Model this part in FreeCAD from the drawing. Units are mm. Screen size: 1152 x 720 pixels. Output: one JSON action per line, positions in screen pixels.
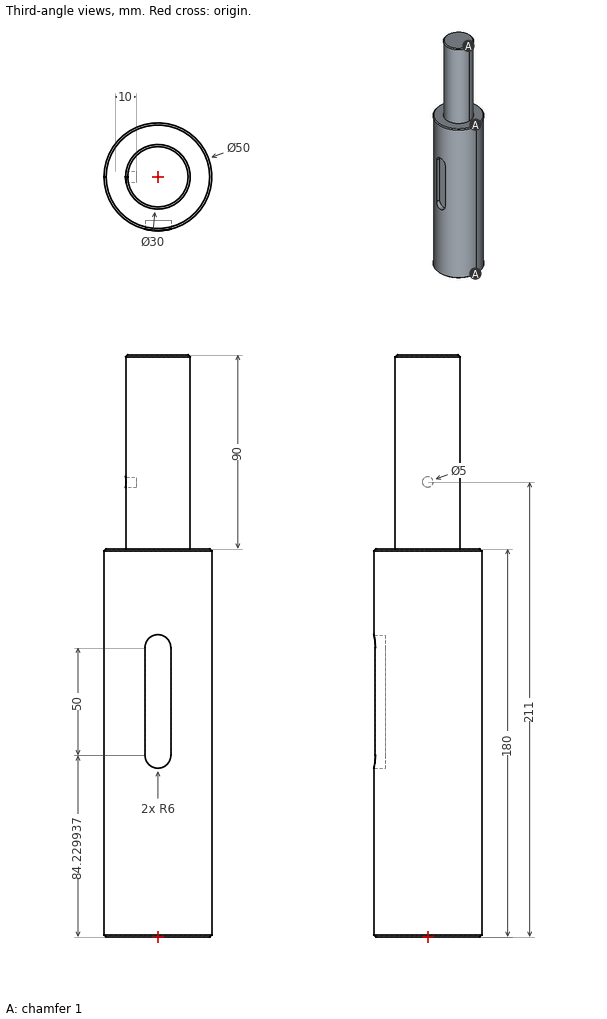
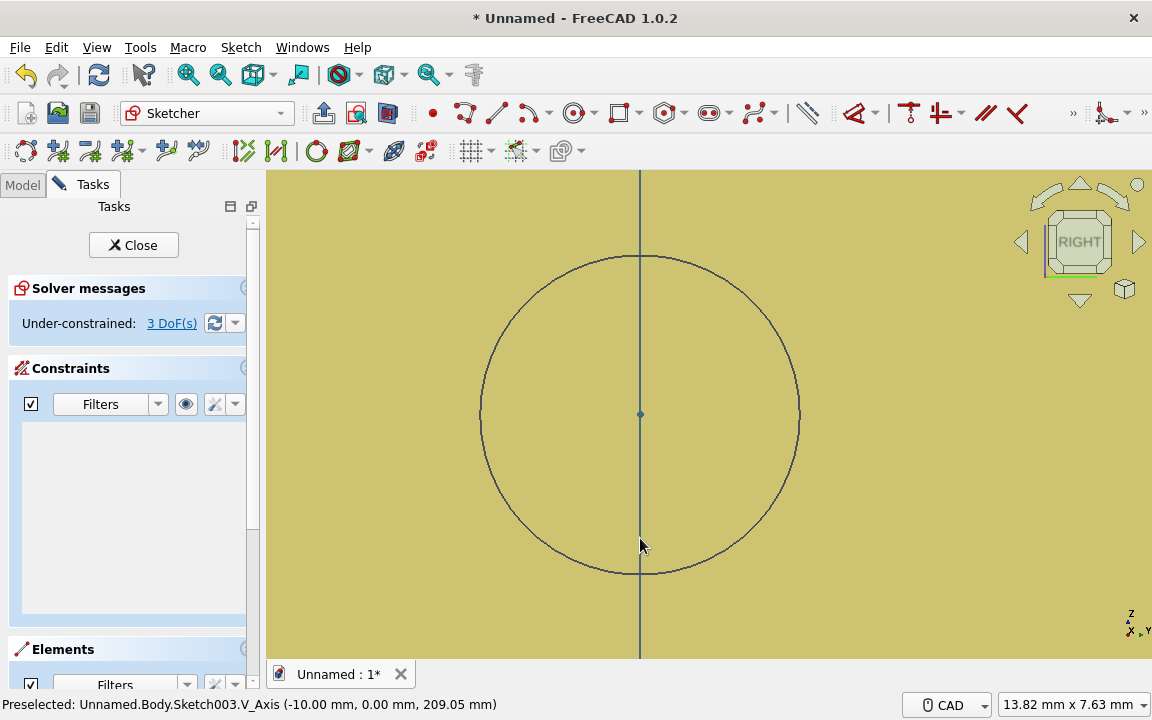
{"action": "left_click", "coordinate": [910, 114]}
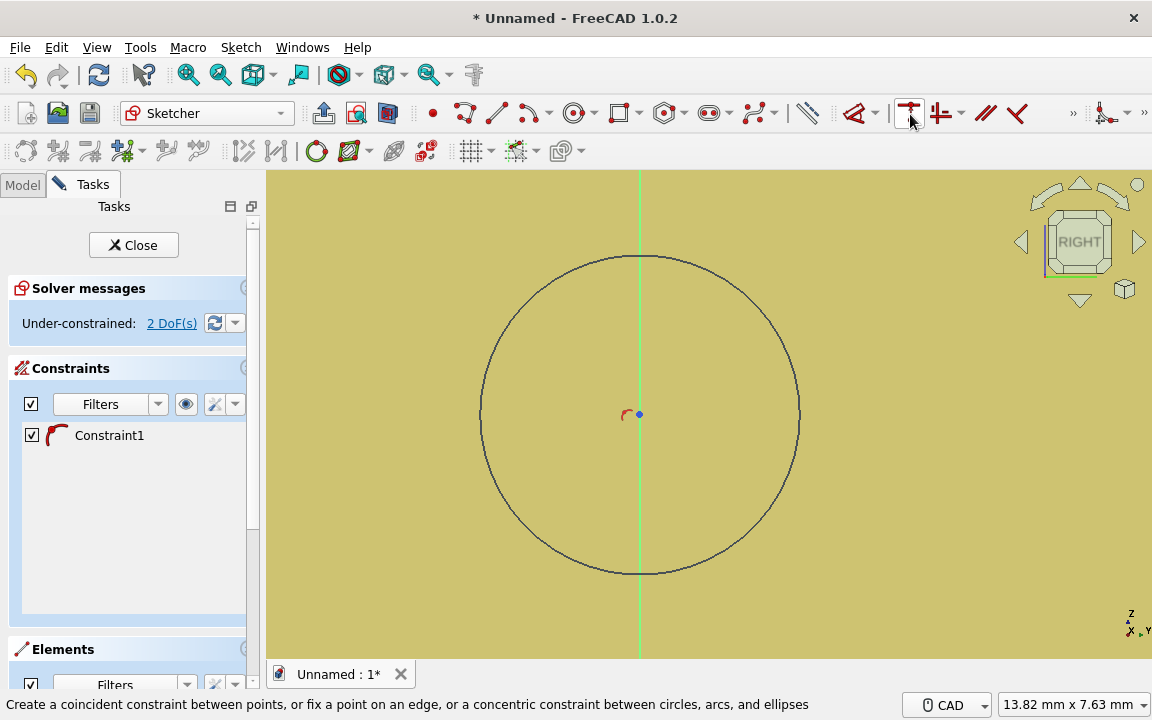
{"action": "key", "text": "d"}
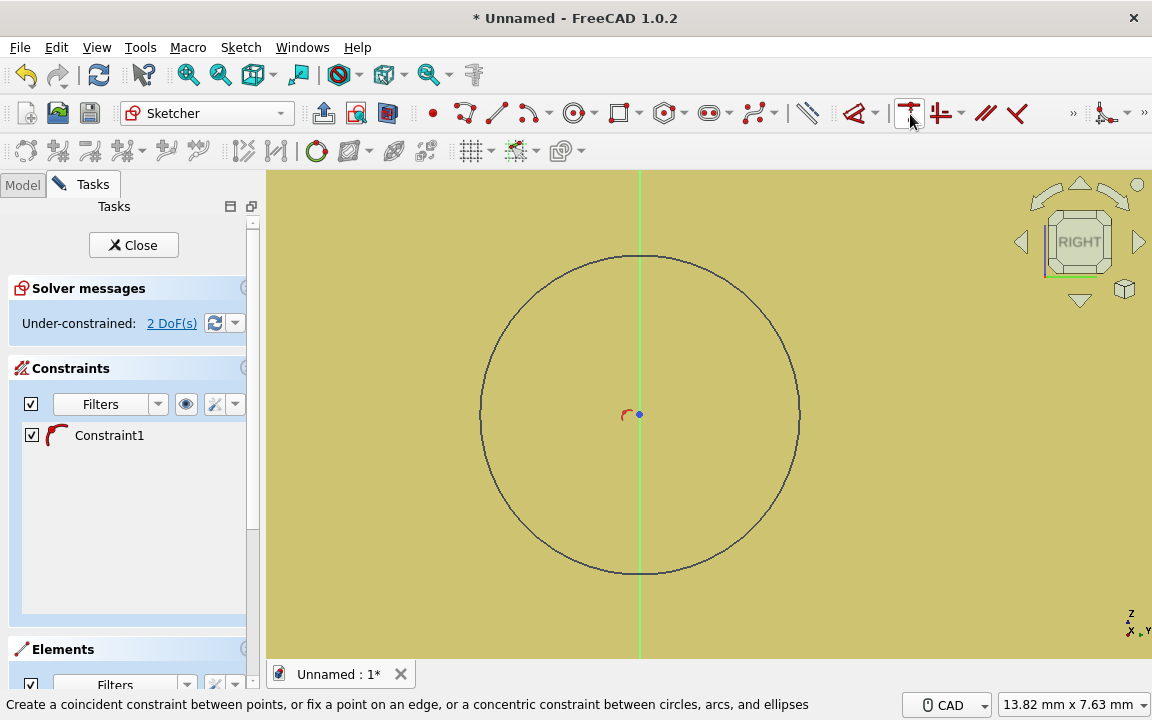
{"action": "left_click", "coordinate": [753, 302]}
{"action": "left_click", "coordinate": [776, 279]}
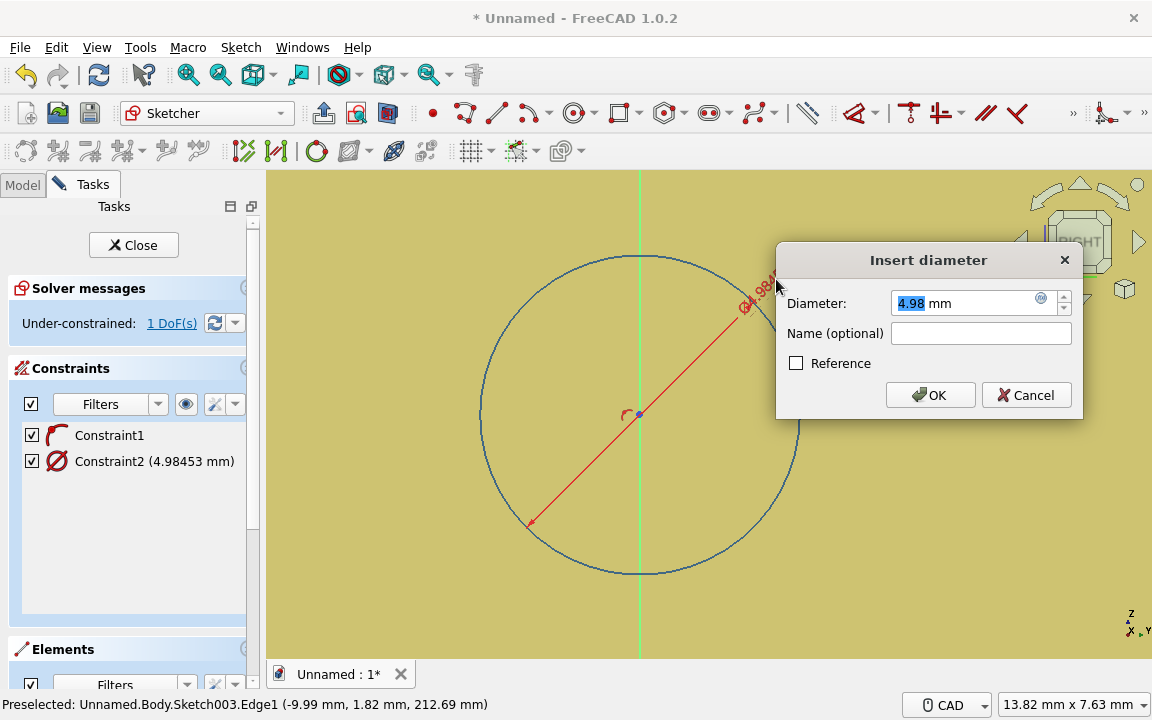
{"action": "type", "text": "5"}
{"action": "key", "text": "Return"}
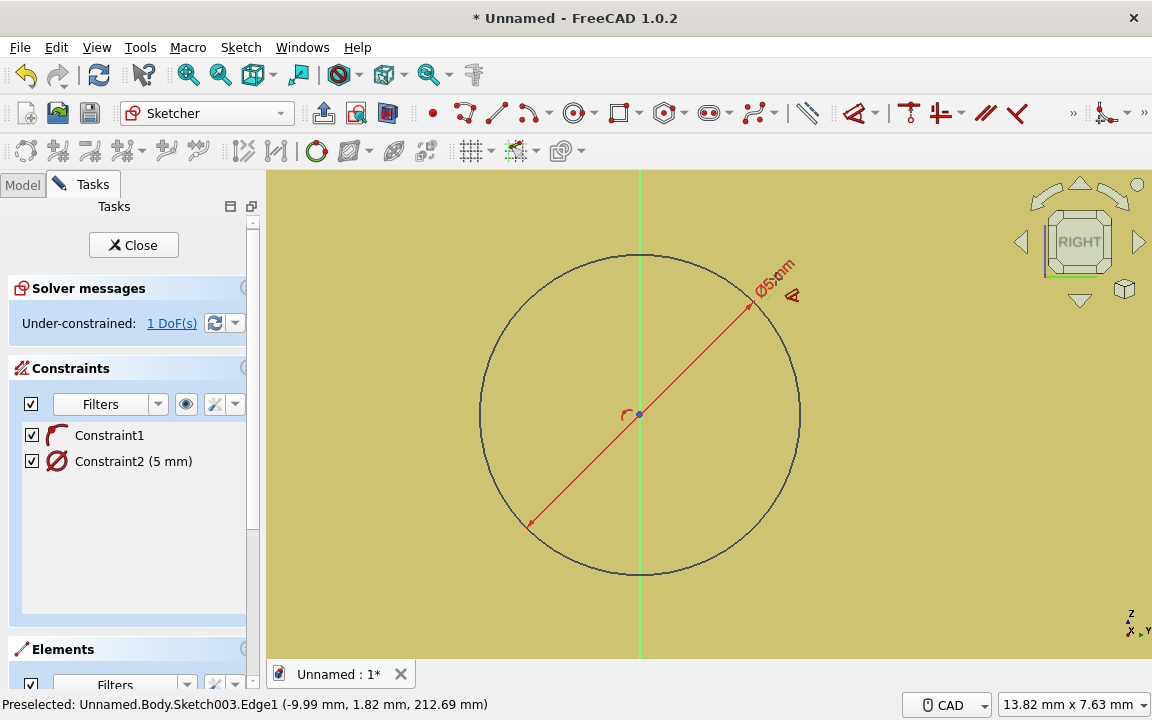
{"action": "left_click", "coordinate": [640, 415]}
{"action": "left_click", "coordinate": [674, 523]}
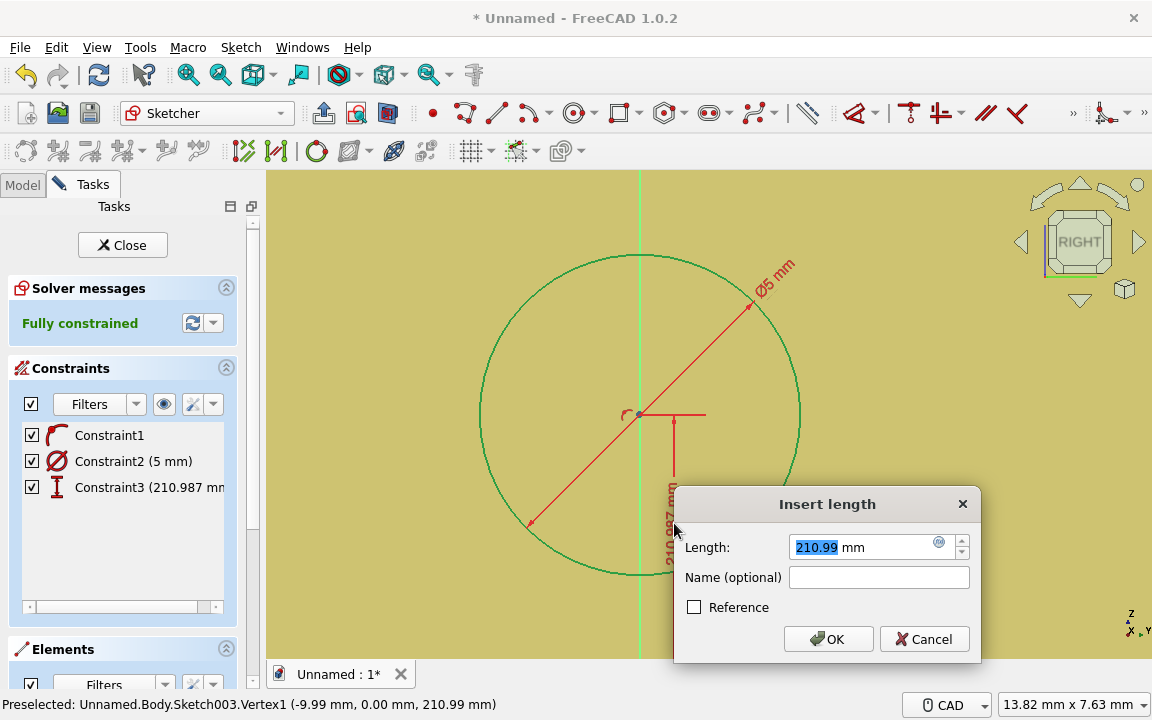
{"action": "type", "text": "211"}
{"action": "key", "text": "Return"}
{"action": "key", "text": "Escape"}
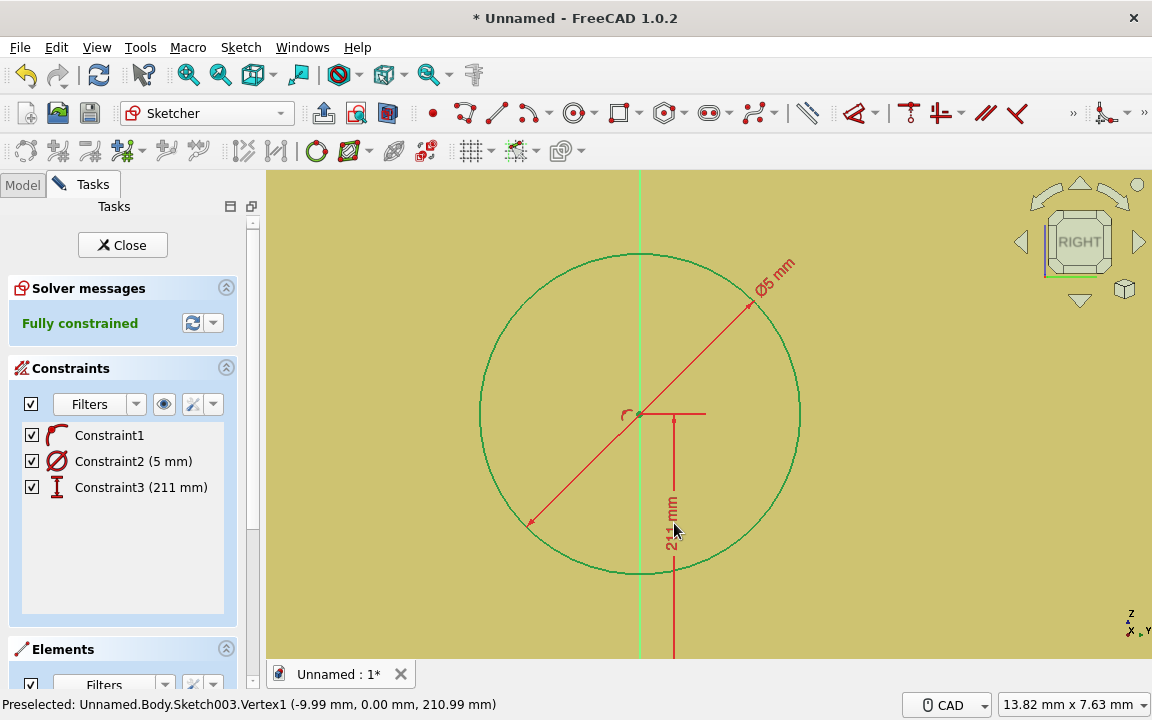
{"action": "left_click", "coordinate": [123, 245]}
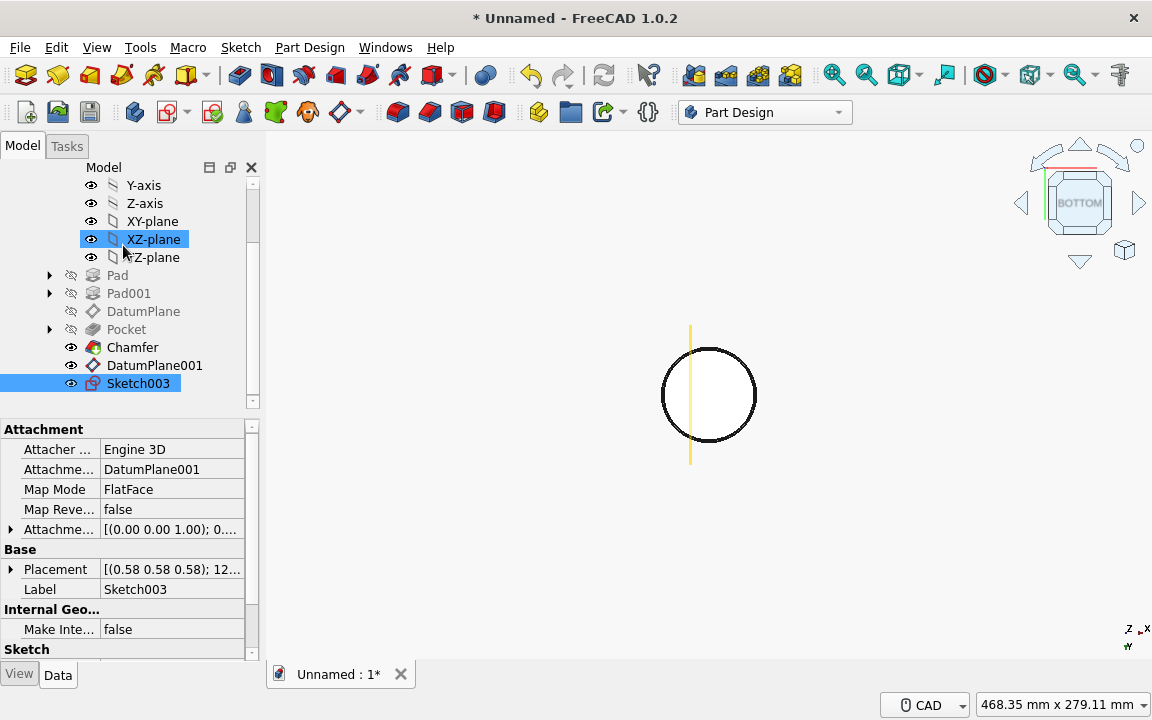
{"action": "left_click", "coordinate": [240, 76]}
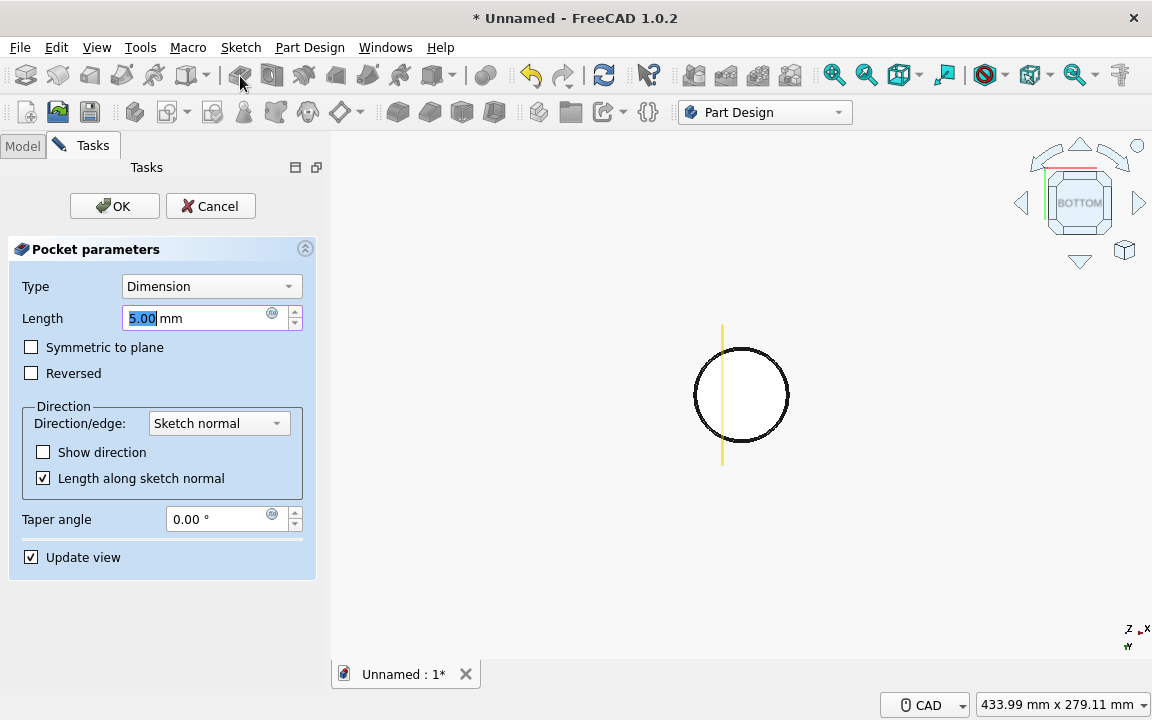
{"action": "type", "text": "10"}
{"action": "key", "text": "Tab"}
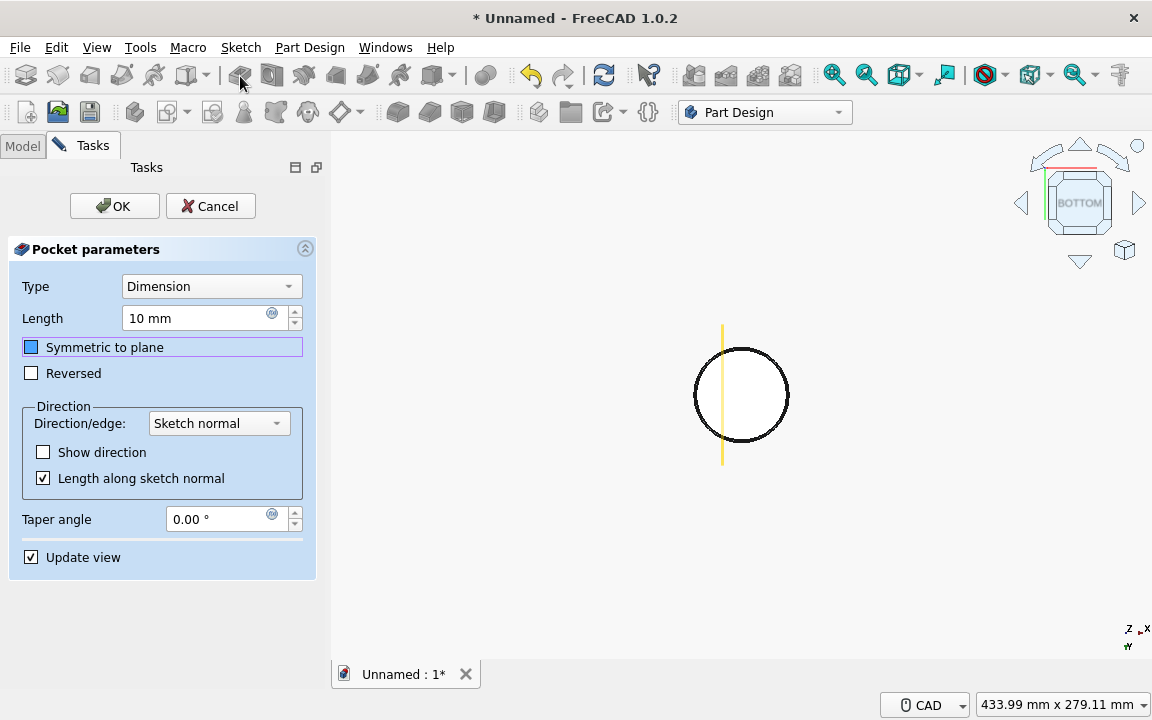
{"action": "left_click", "coordinate": [115, 206]}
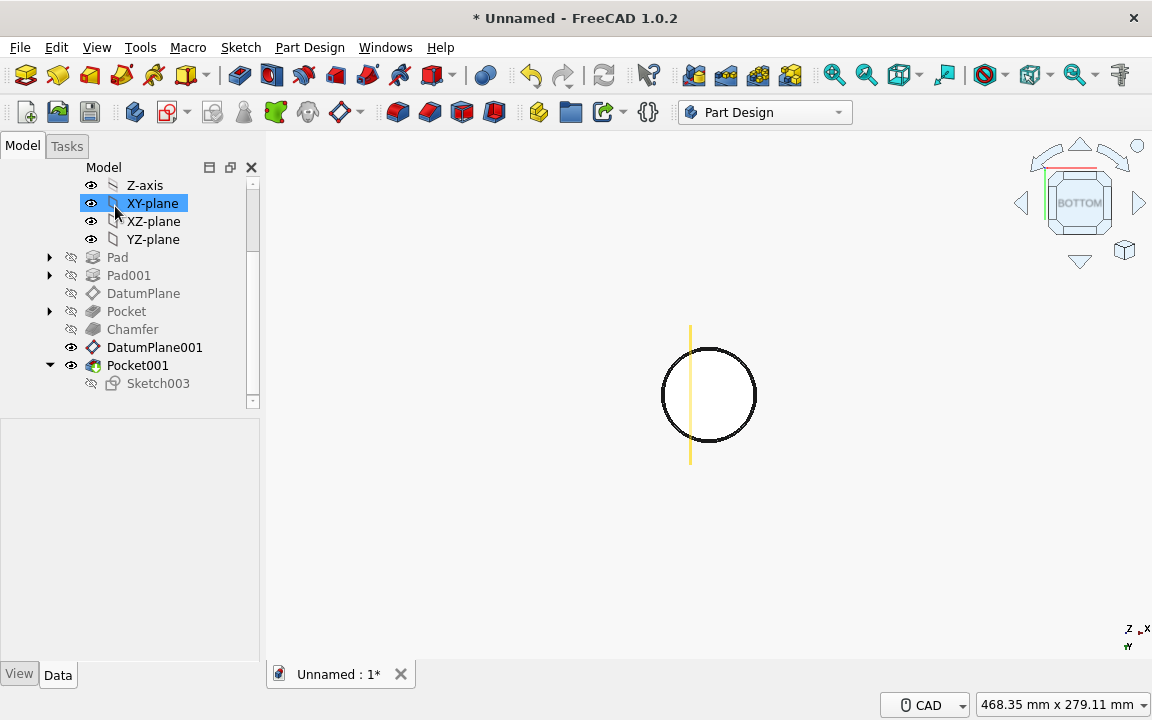
{"action": "left_click", "coordinate": [116, 347]}
{"action": "key", "text": "space"}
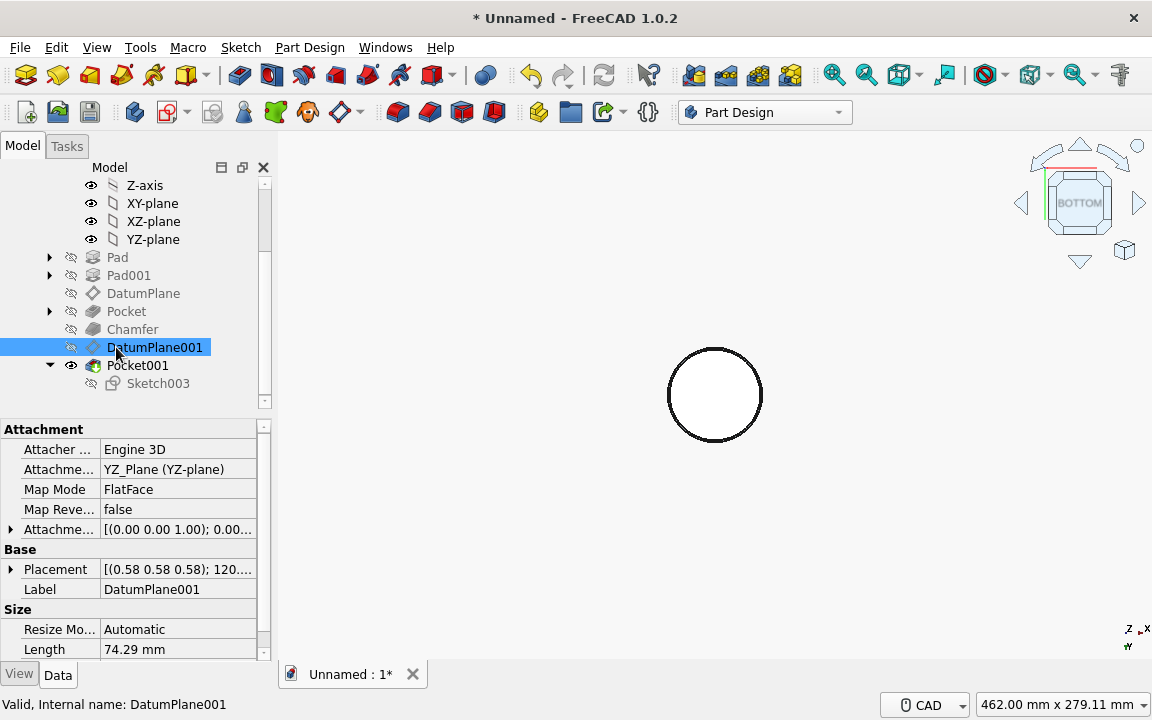
{"action": "key", "text": "0"}